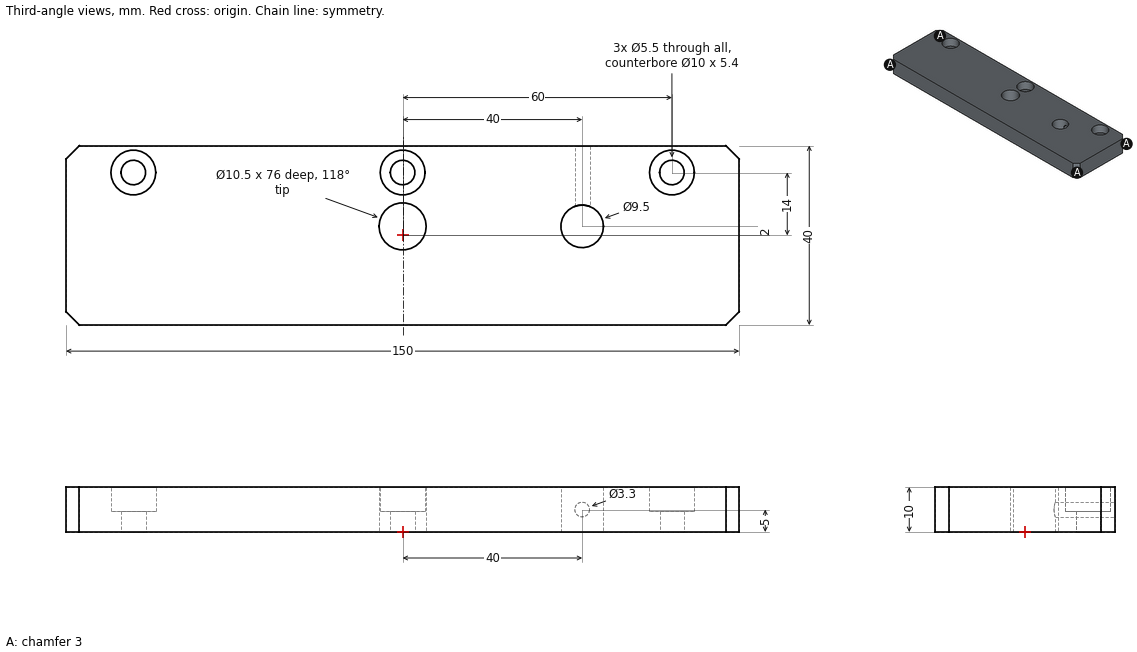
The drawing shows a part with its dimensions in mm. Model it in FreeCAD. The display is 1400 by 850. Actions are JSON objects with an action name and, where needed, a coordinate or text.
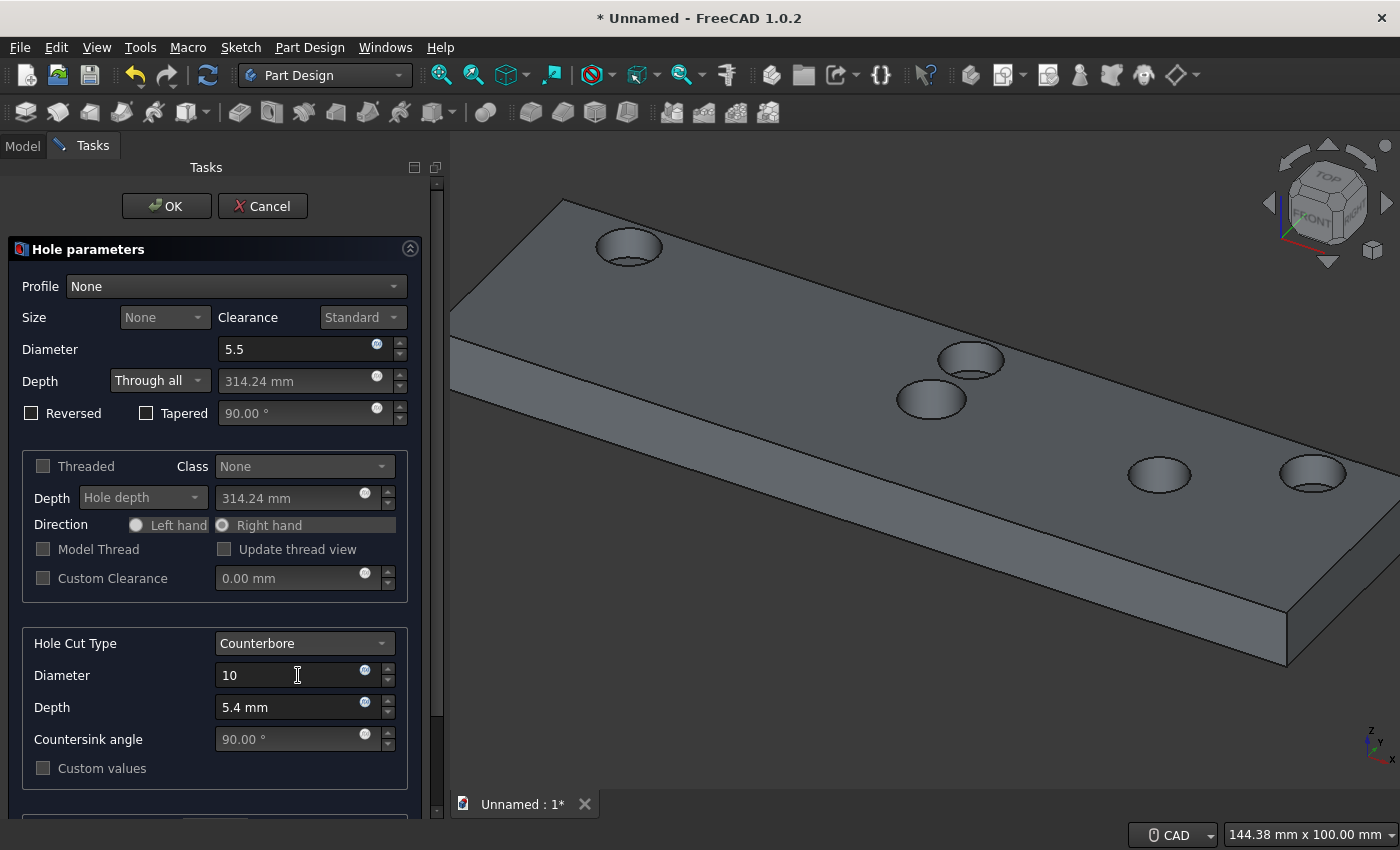
{"action": "left_click", "coordinate": [167, 206]}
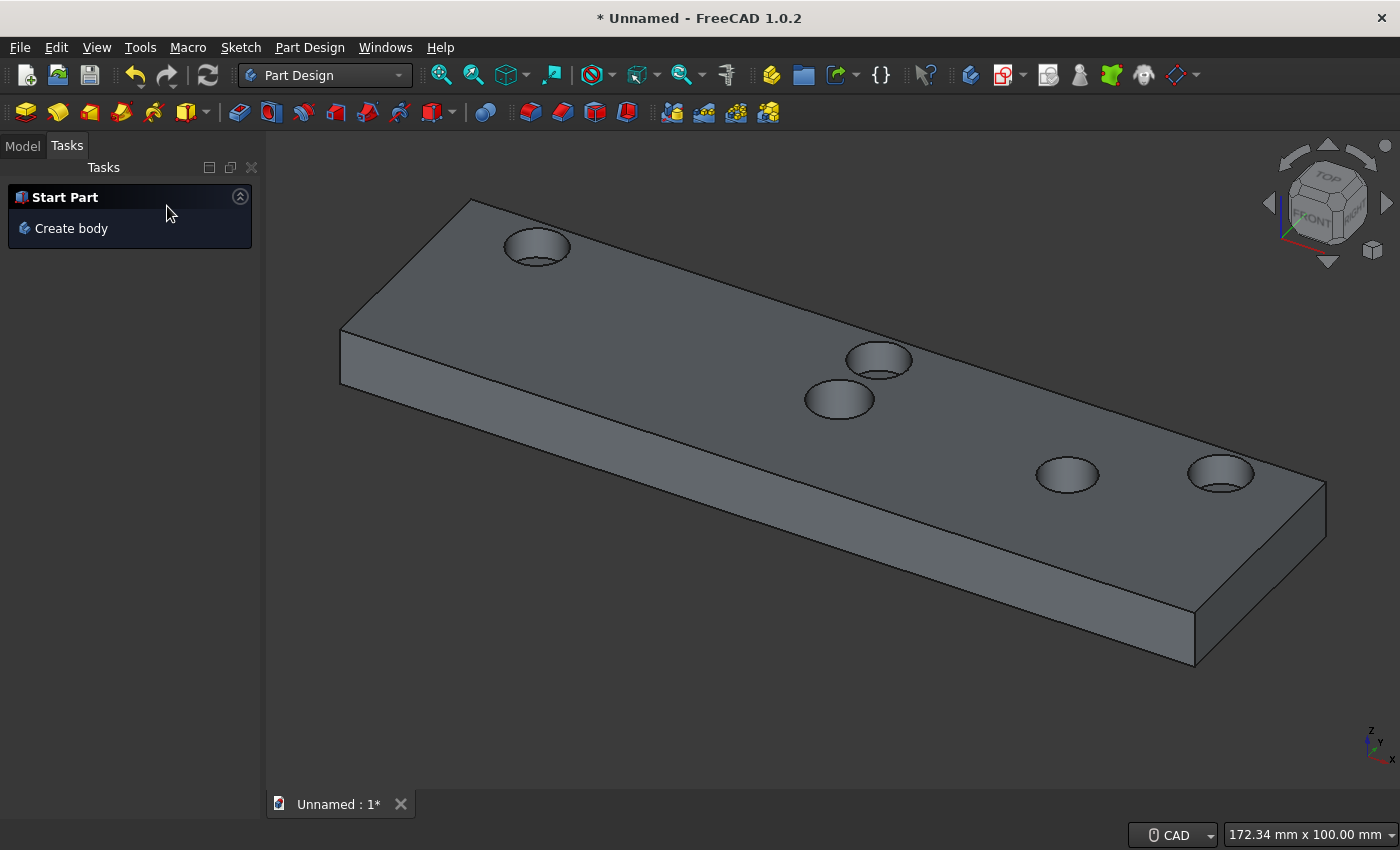
{"action": "key", "text": "4"}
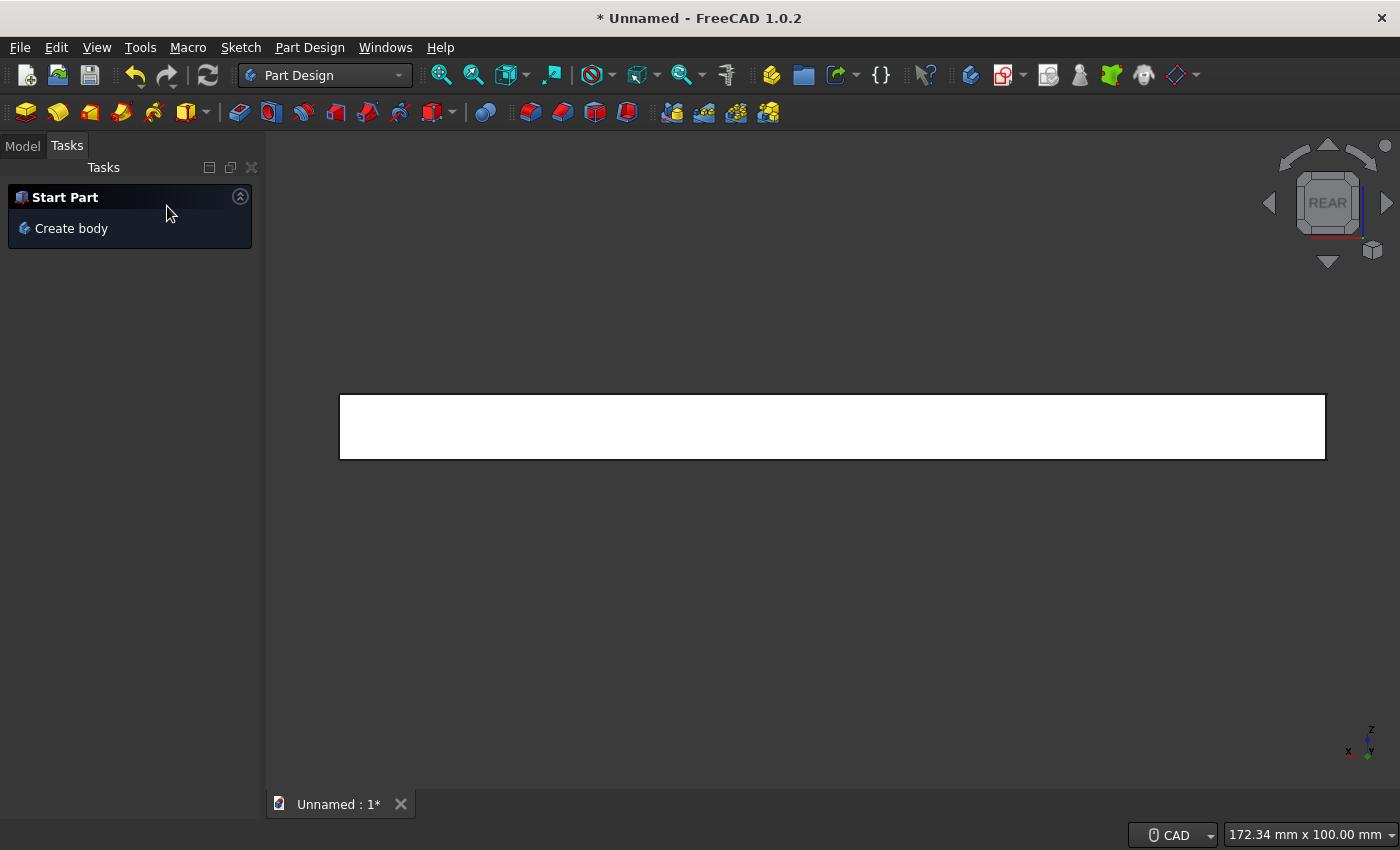
{"action": "left_click", "coordinate": [410, 426]}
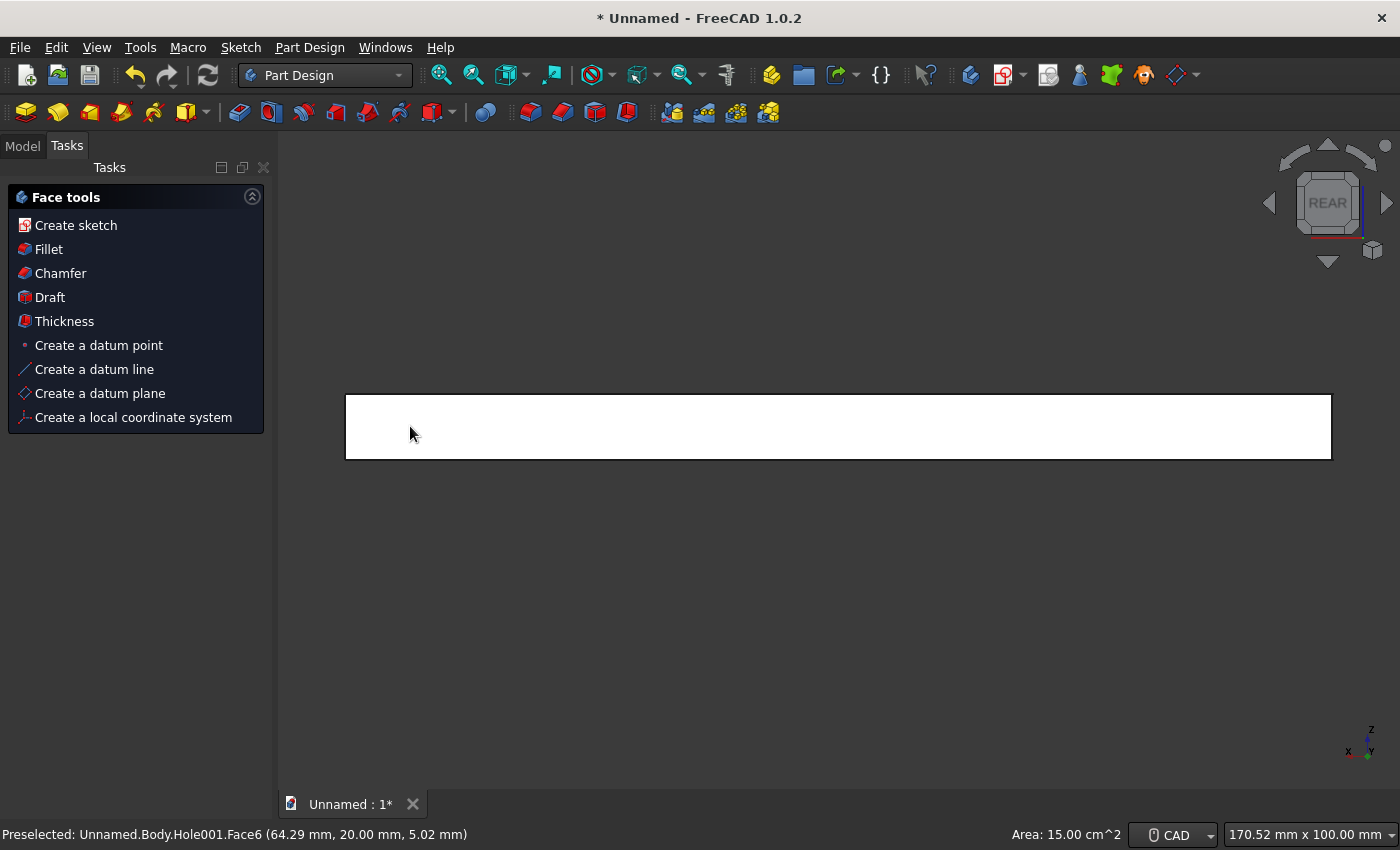
{"action": "left_click", "coordinate": [1004, 76]}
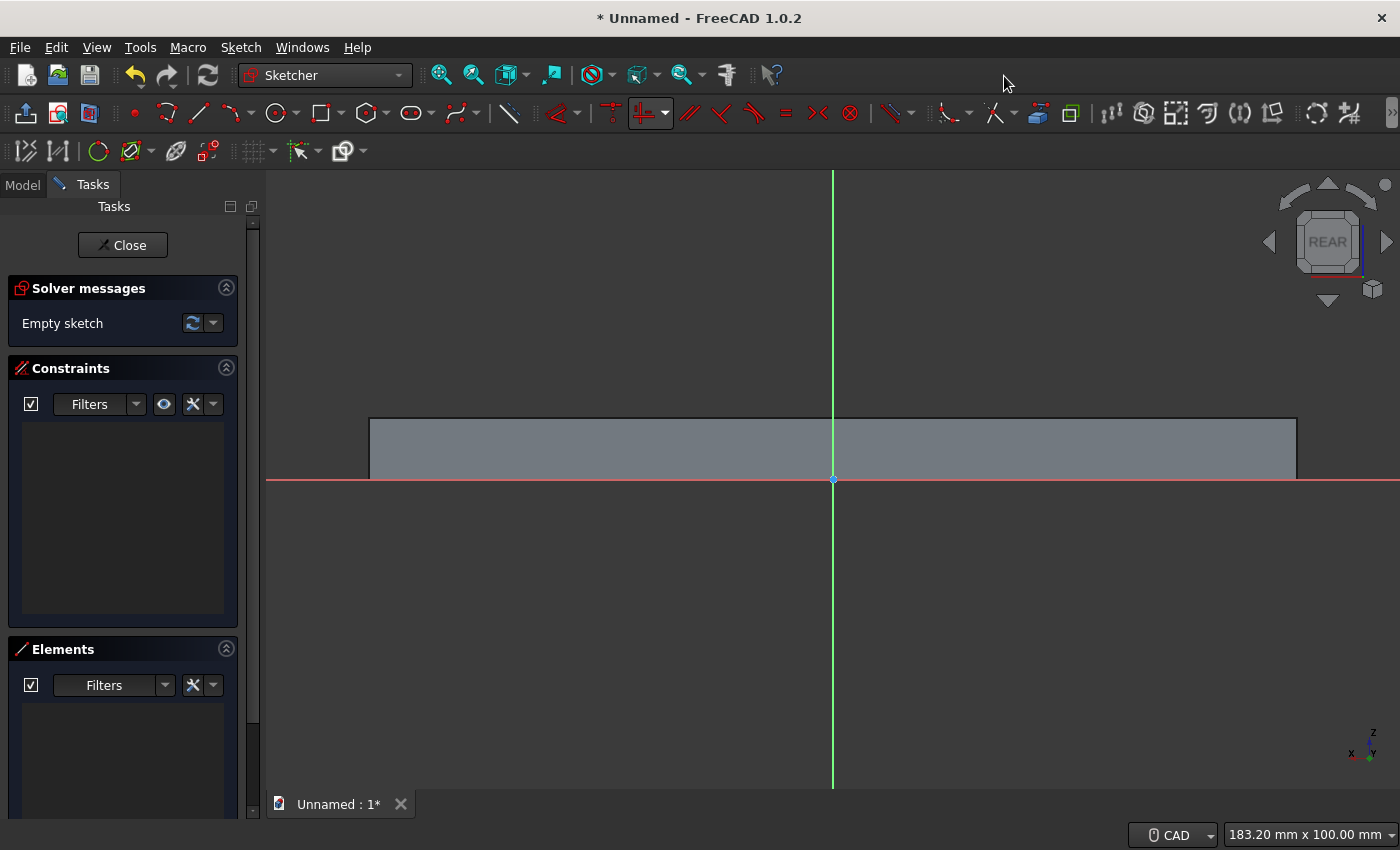
{"action": "scroll", "coordinate": [576, 447], "scroll_direction": "up", "scroll_amount": 15}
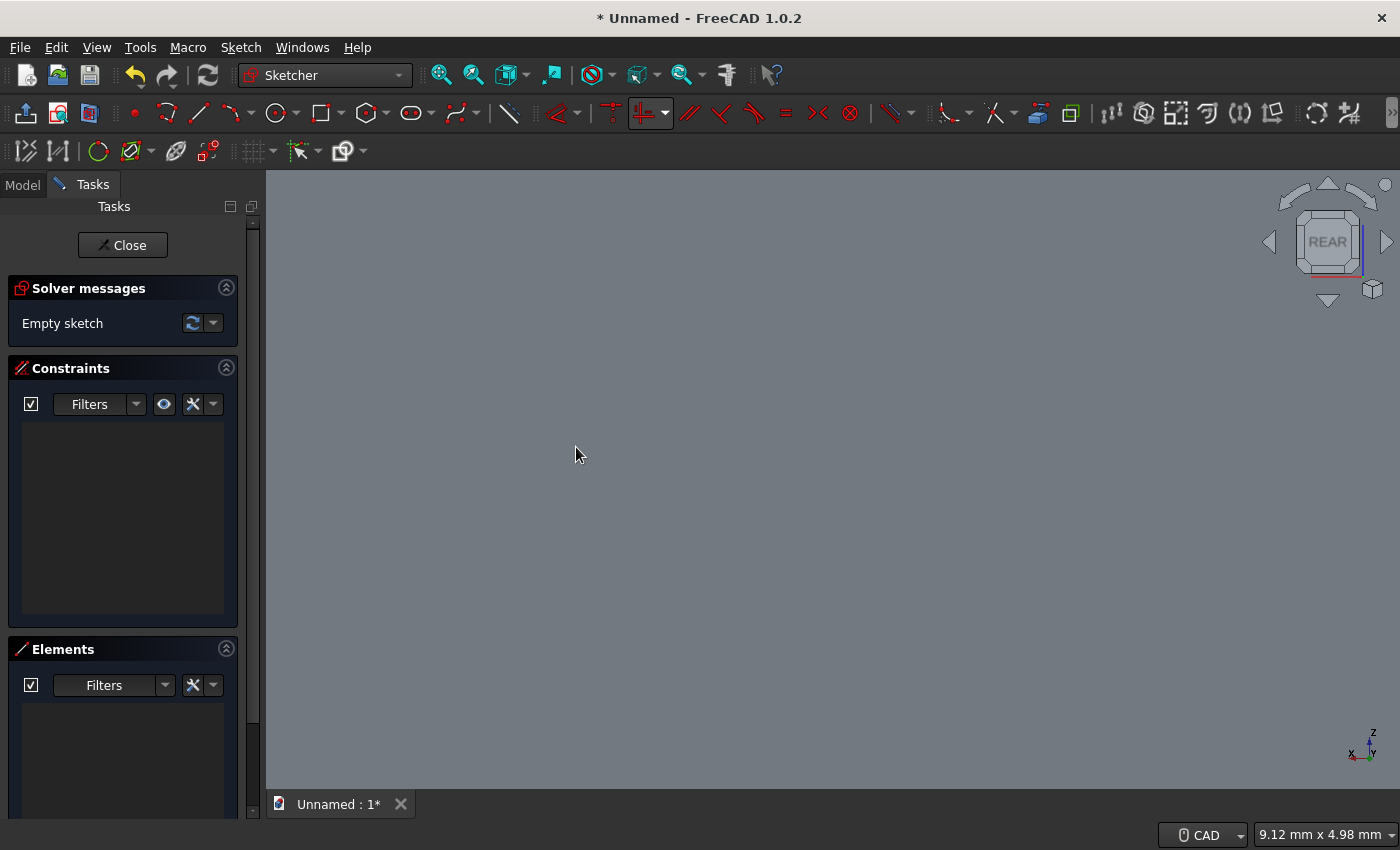
{"action": "key", "text": "g c"}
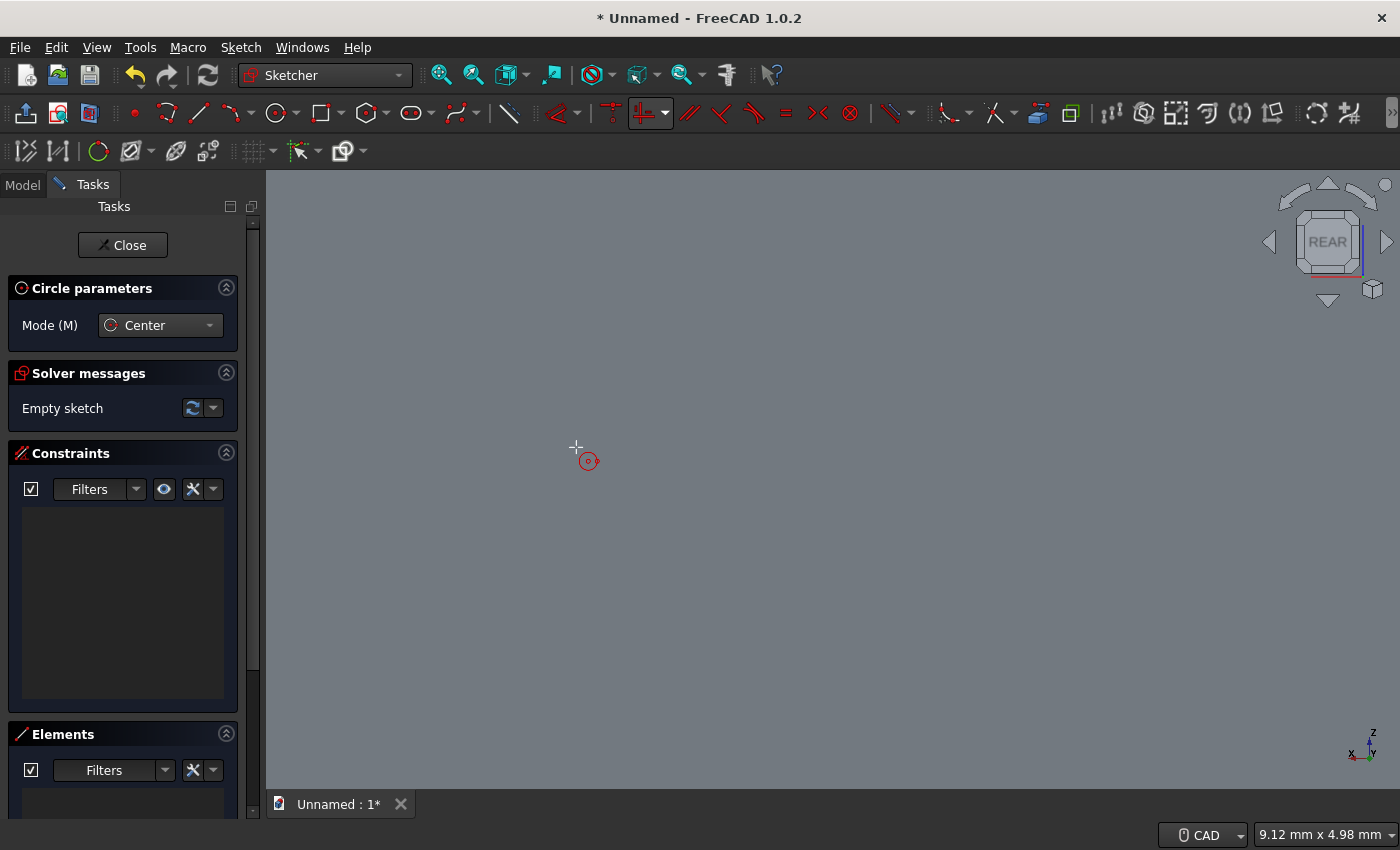
{"action": "left_click", "coordinate": [760, 470]}
{"action": "mouse_move", "coordinate": [905, 325]}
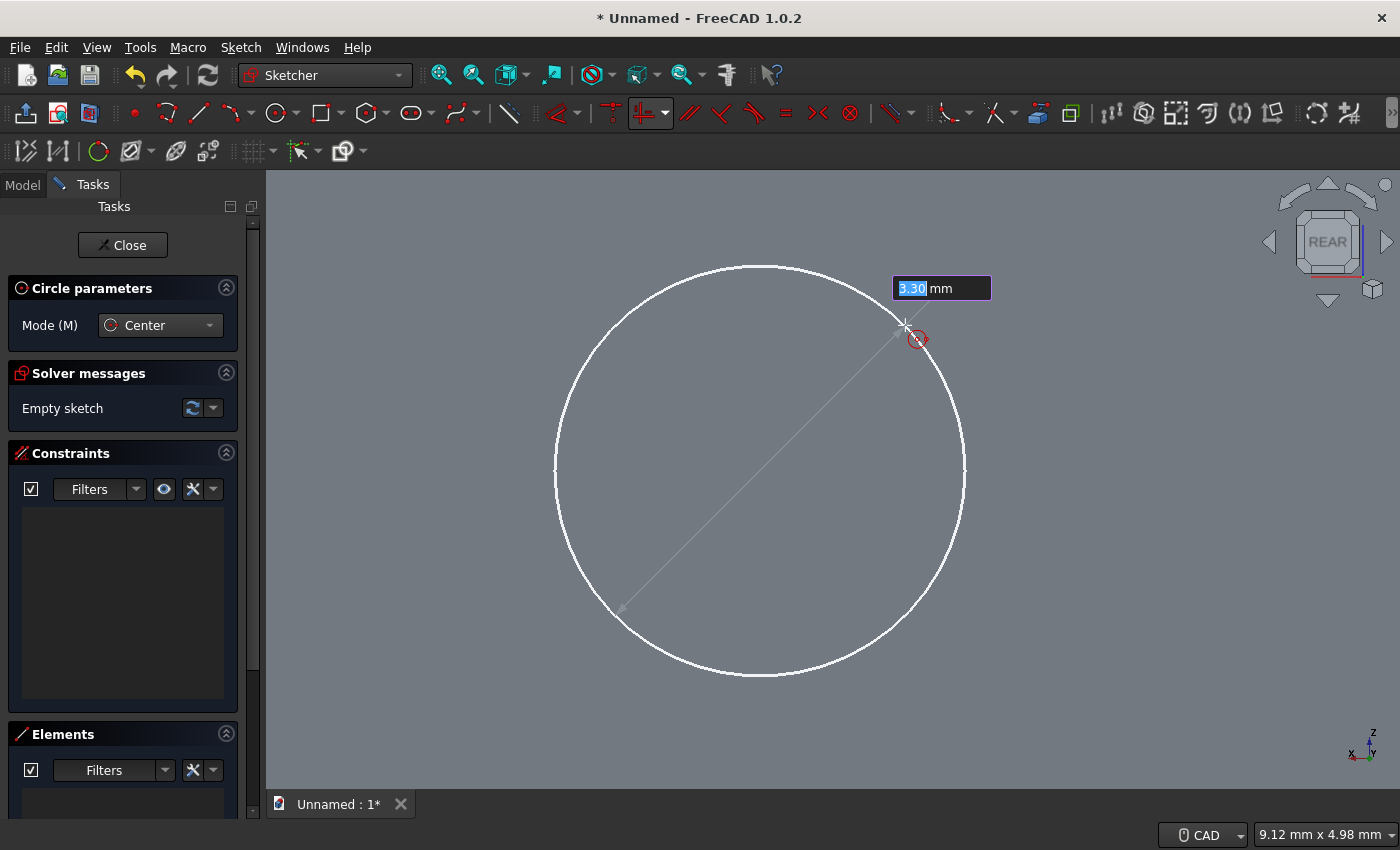
{"action": "type", "text": "3.3"}
{"action": "key", "text": "Return"}
{"action": "key", "text": "Escape"}